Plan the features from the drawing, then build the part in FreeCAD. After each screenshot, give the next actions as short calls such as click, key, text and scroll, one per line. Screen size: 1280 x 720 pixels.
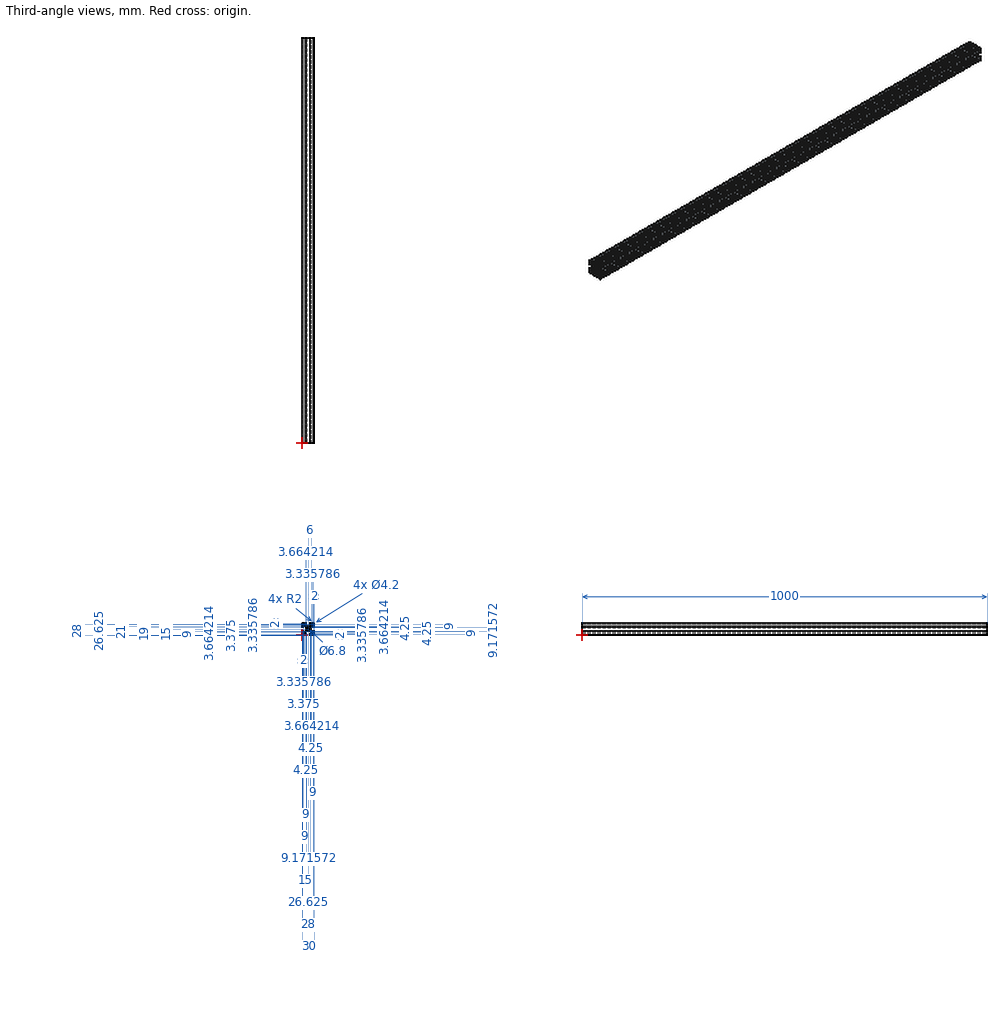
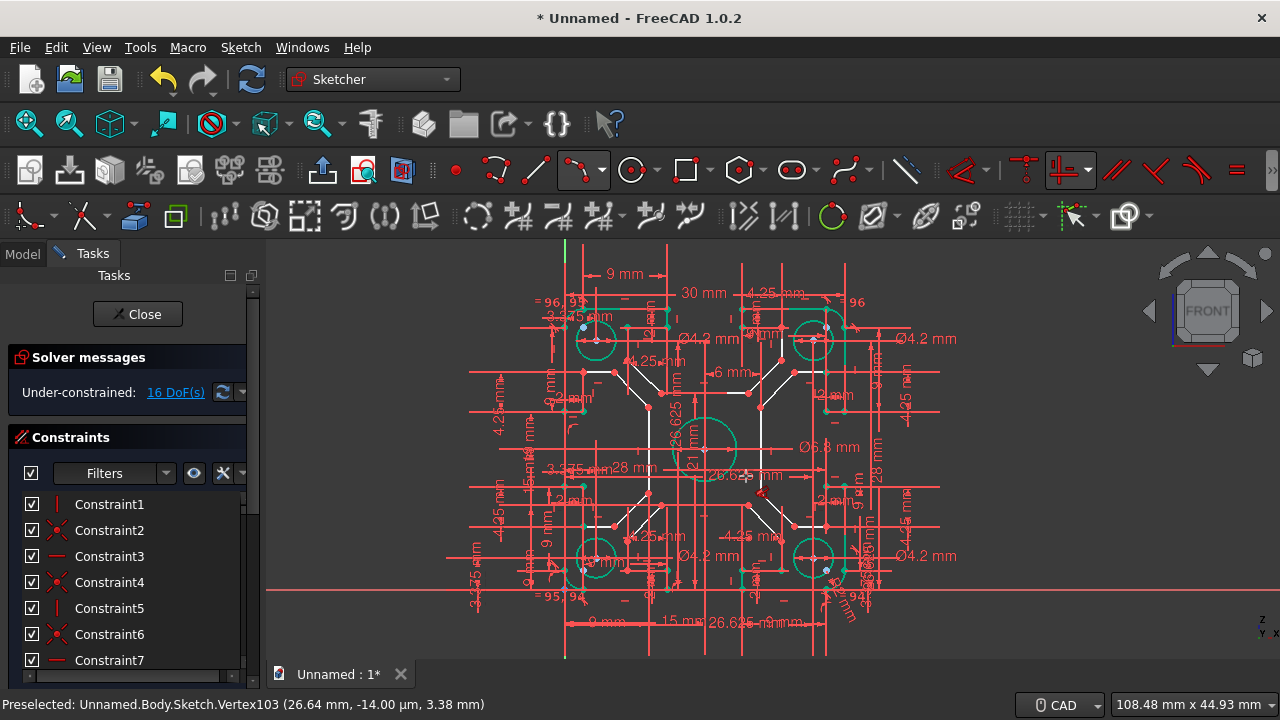
scroll(817, 372, up, 2)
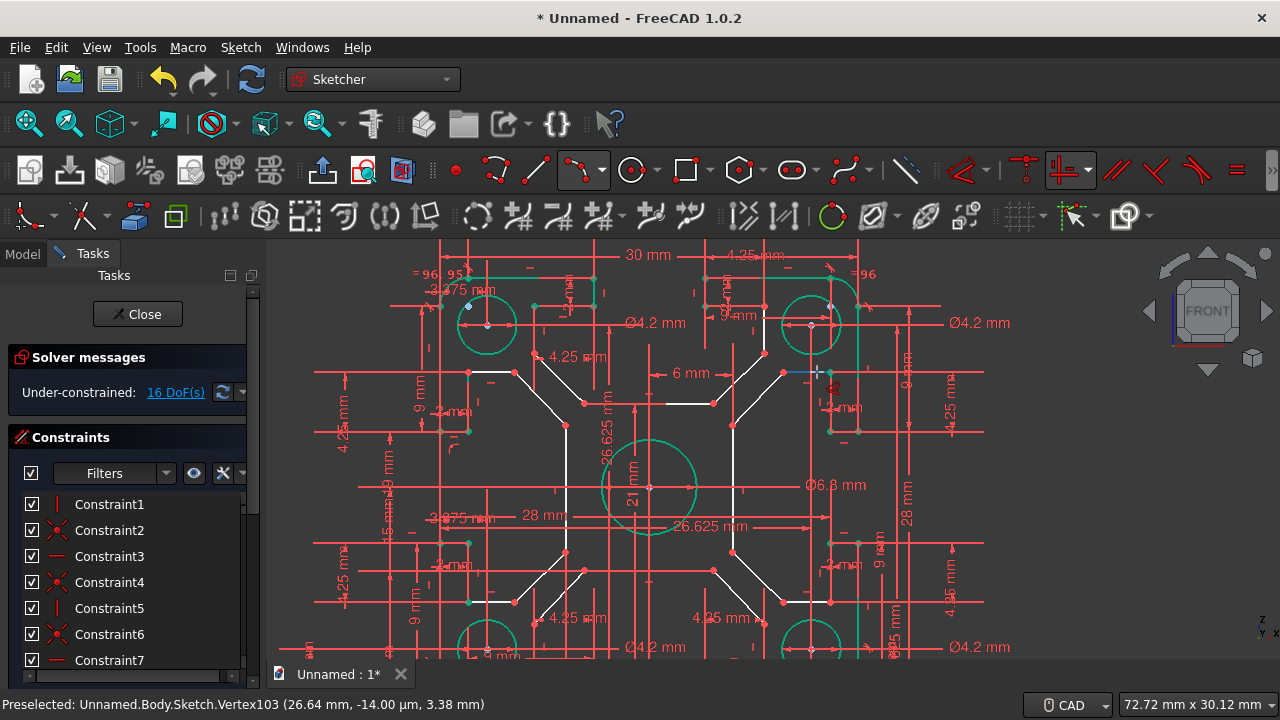
click(816, 372)
click(807, 338)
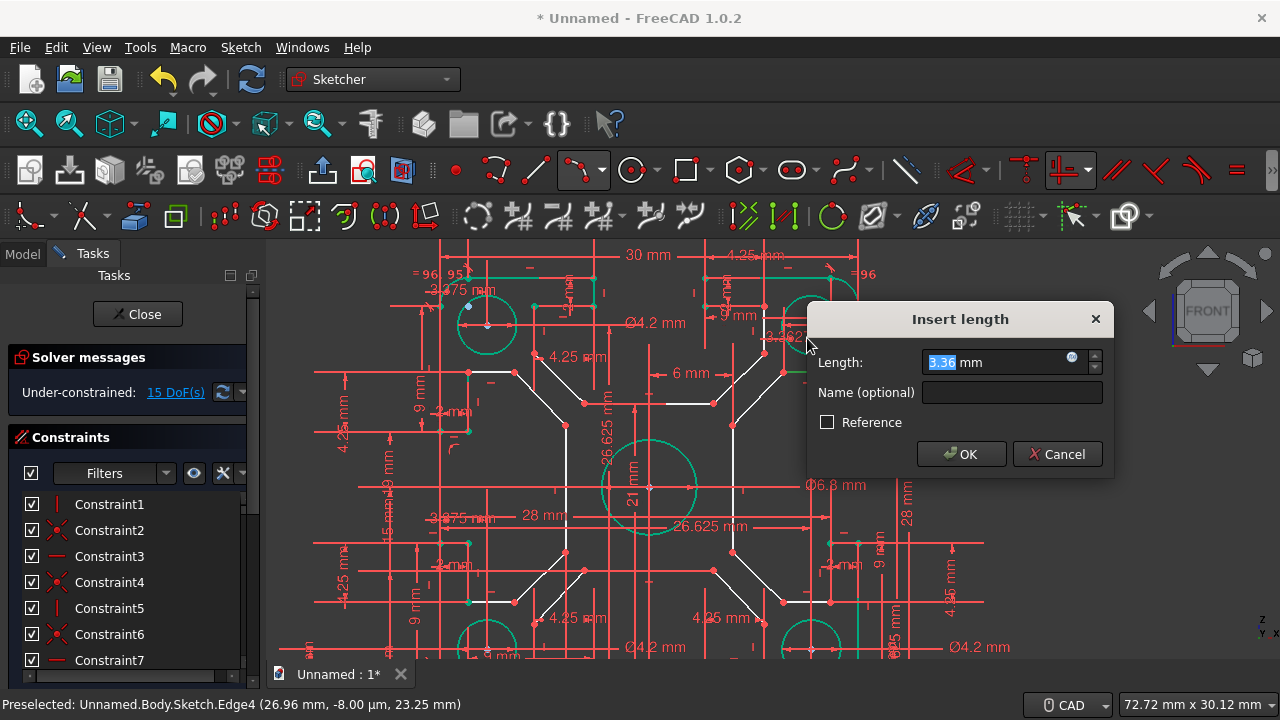
text(3.335786)
key(Return)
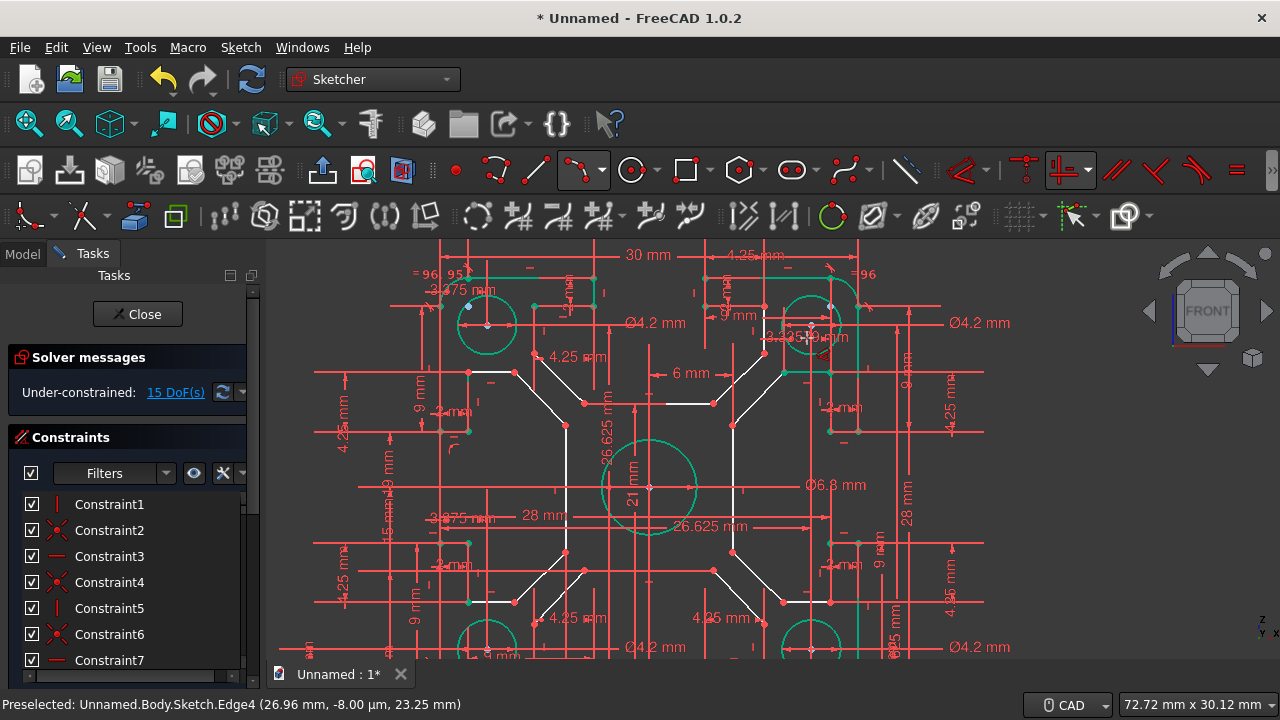
click(733, 464)
click(767, 489)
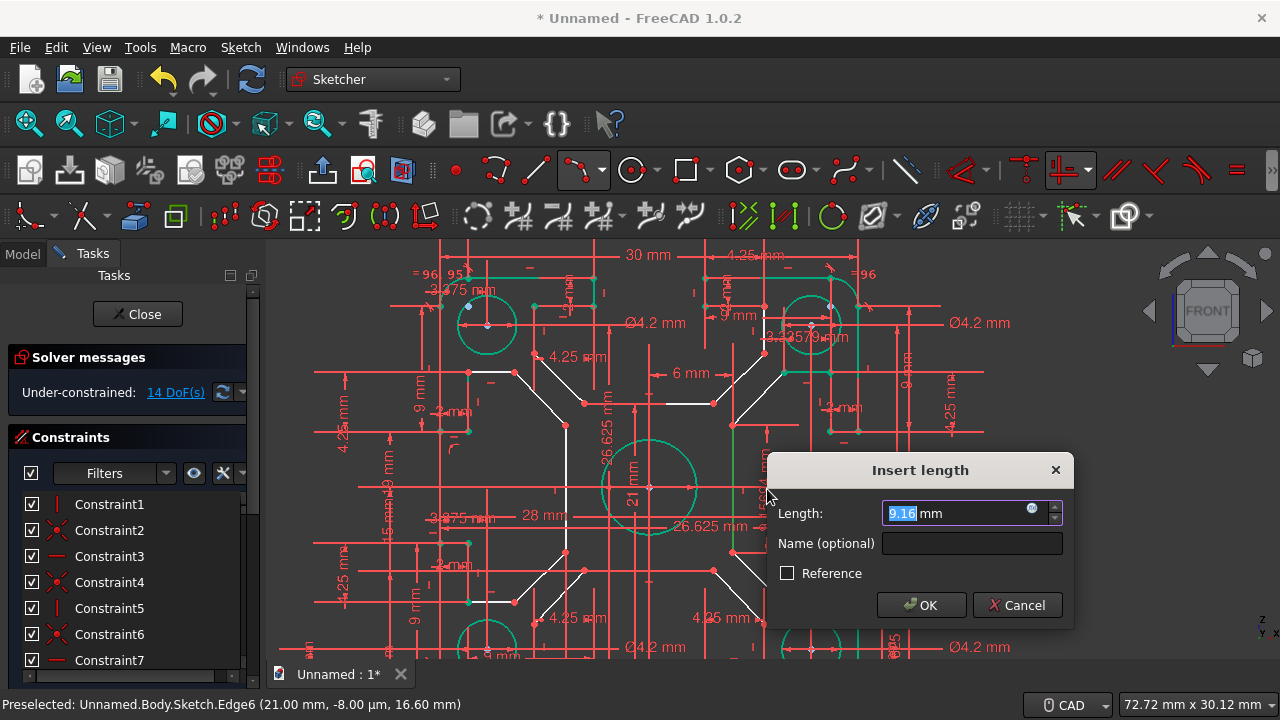
text(9.171572)
key(Return)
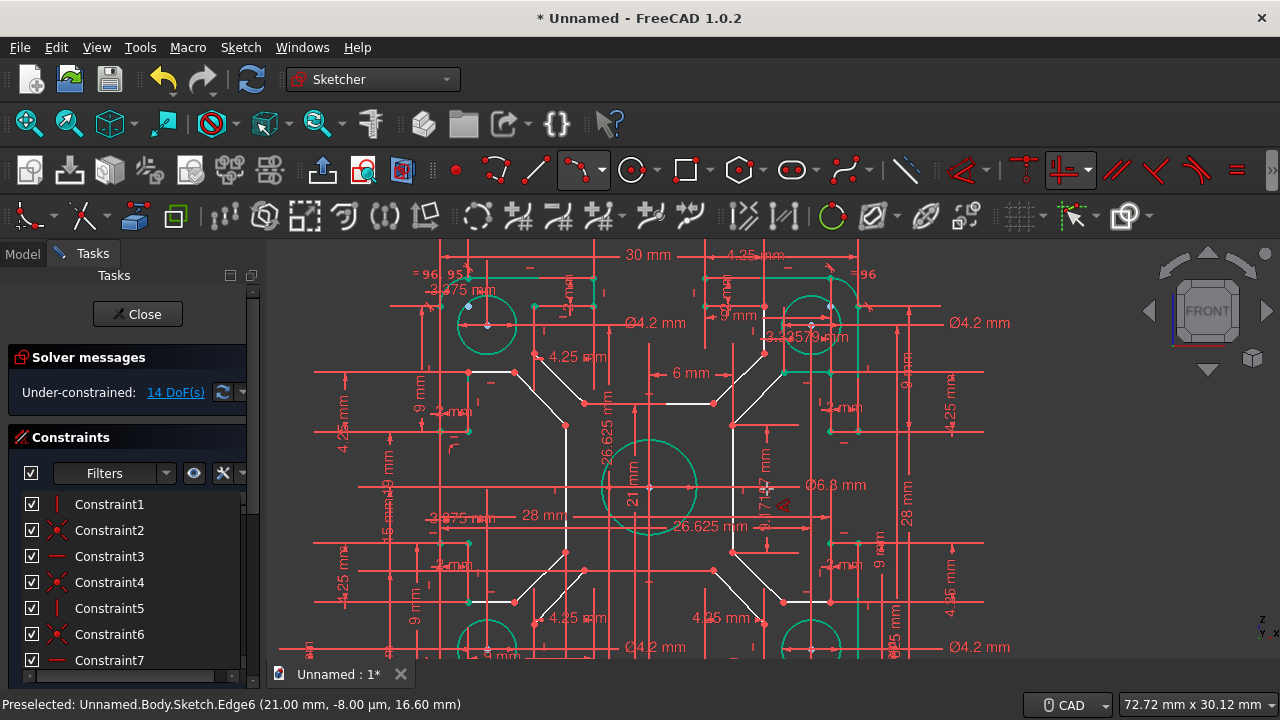
click(798, 602)
click(807, 544)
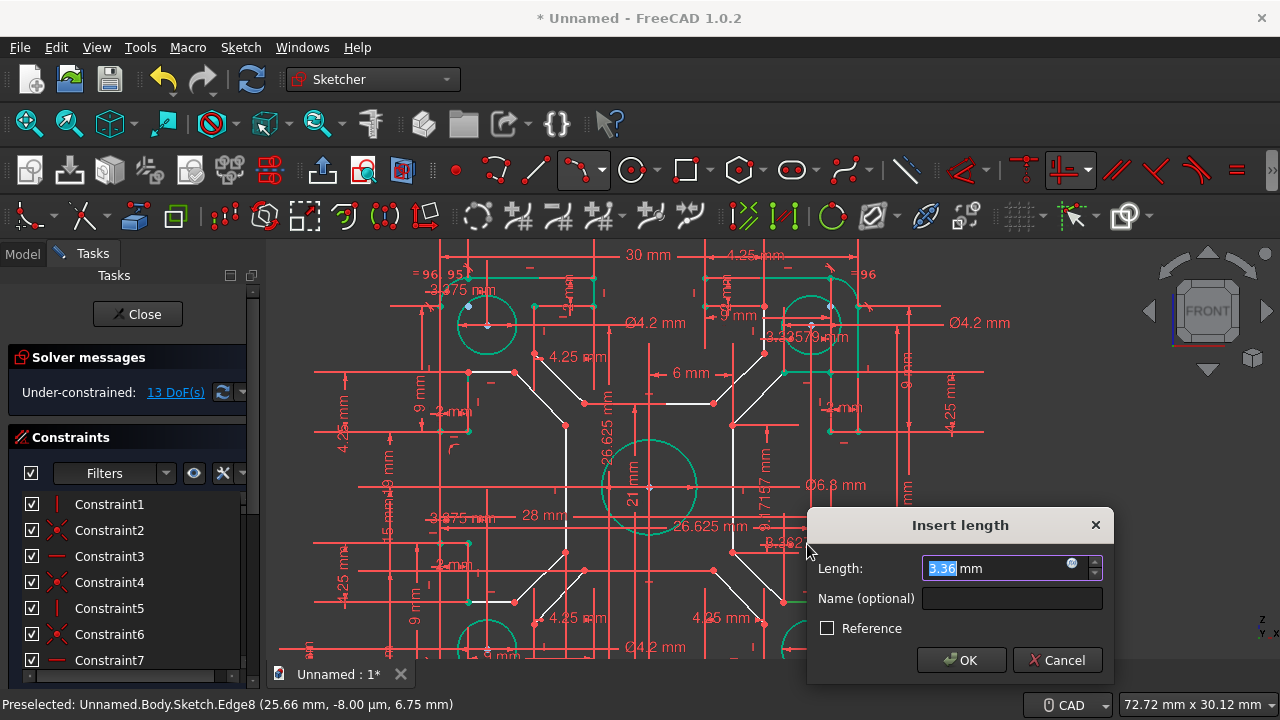
text(3.335786)
key(Return)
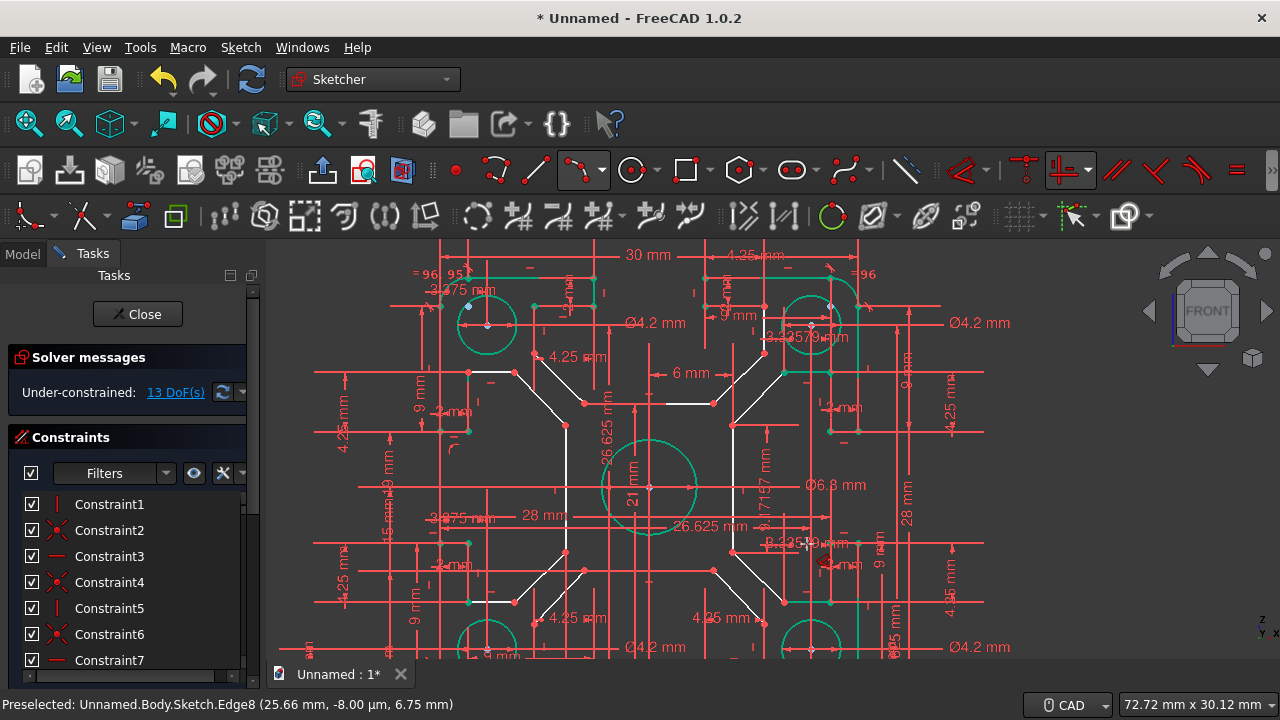
scroll(817, 371, down, 2)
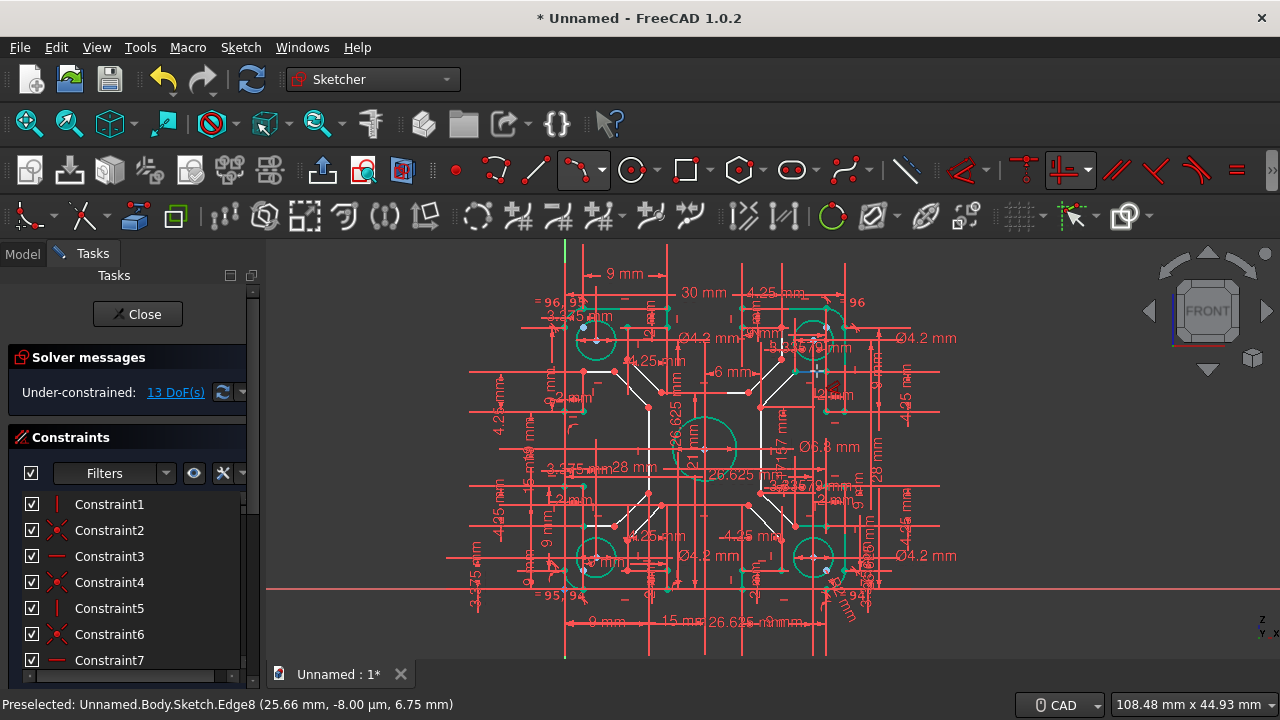
scroll(782, 562, up, 3)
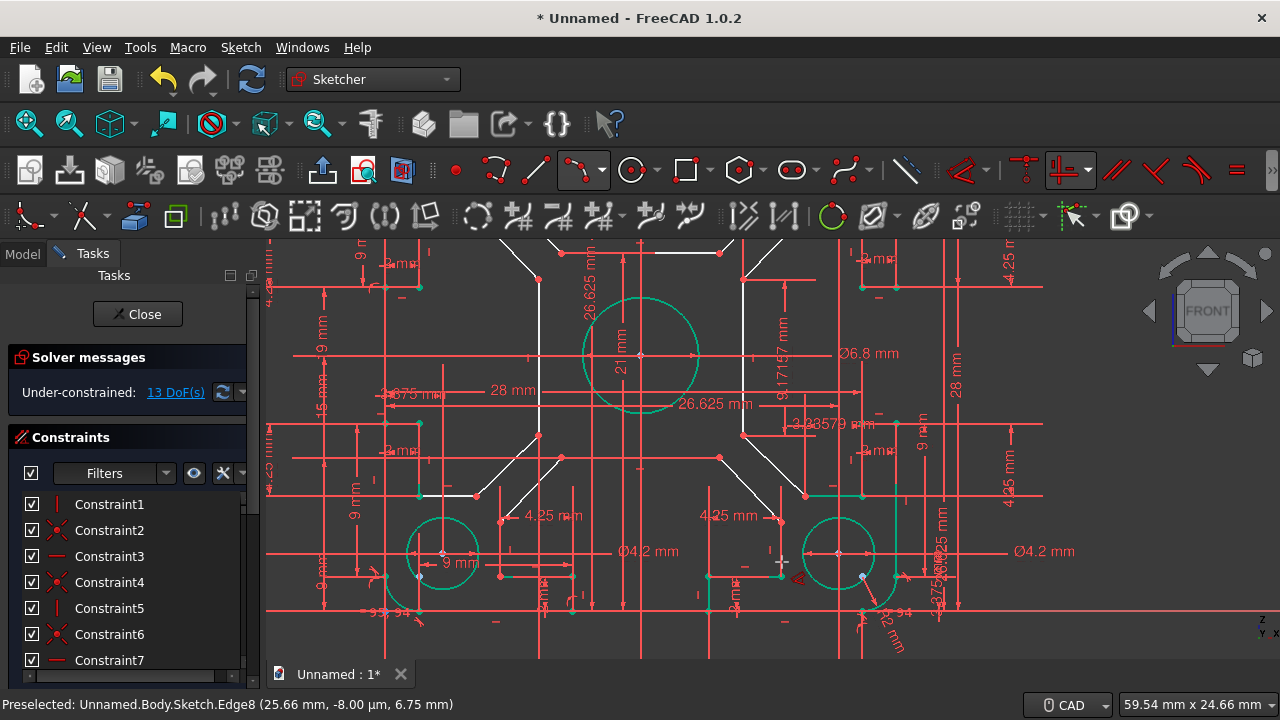
click(781, 561)
click(747, 550)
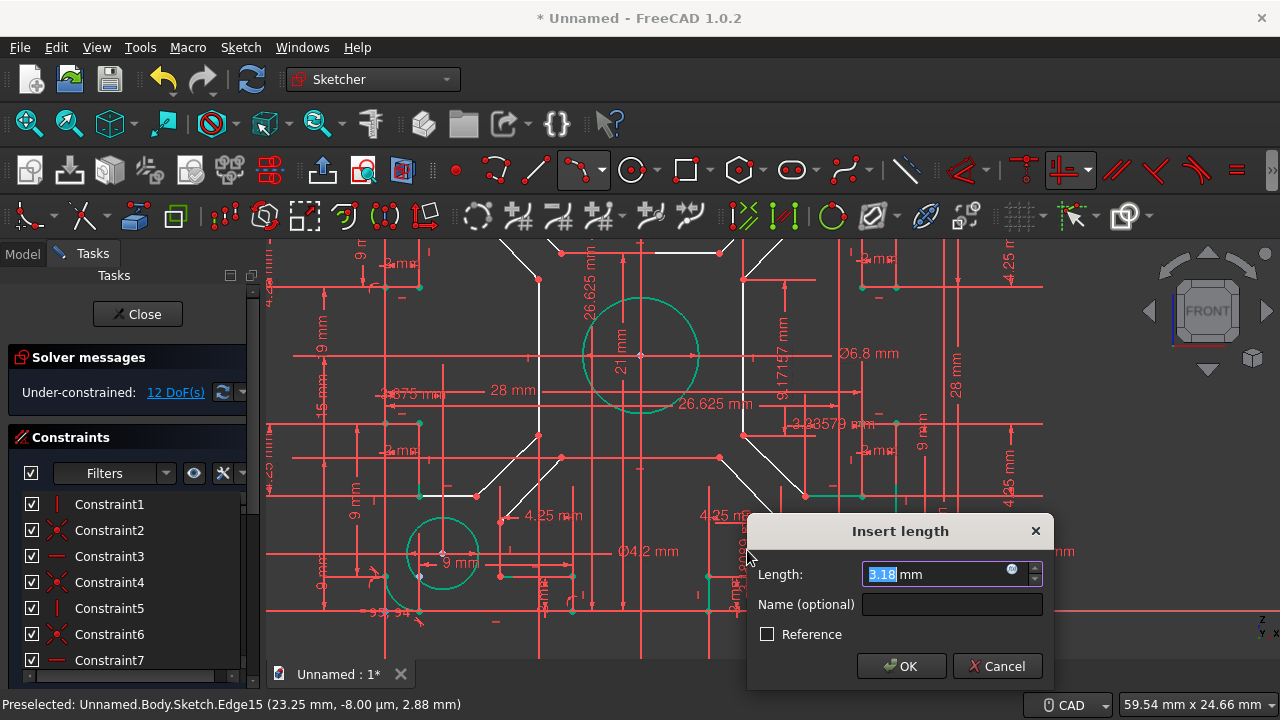
text(3.335786)
key(Return)